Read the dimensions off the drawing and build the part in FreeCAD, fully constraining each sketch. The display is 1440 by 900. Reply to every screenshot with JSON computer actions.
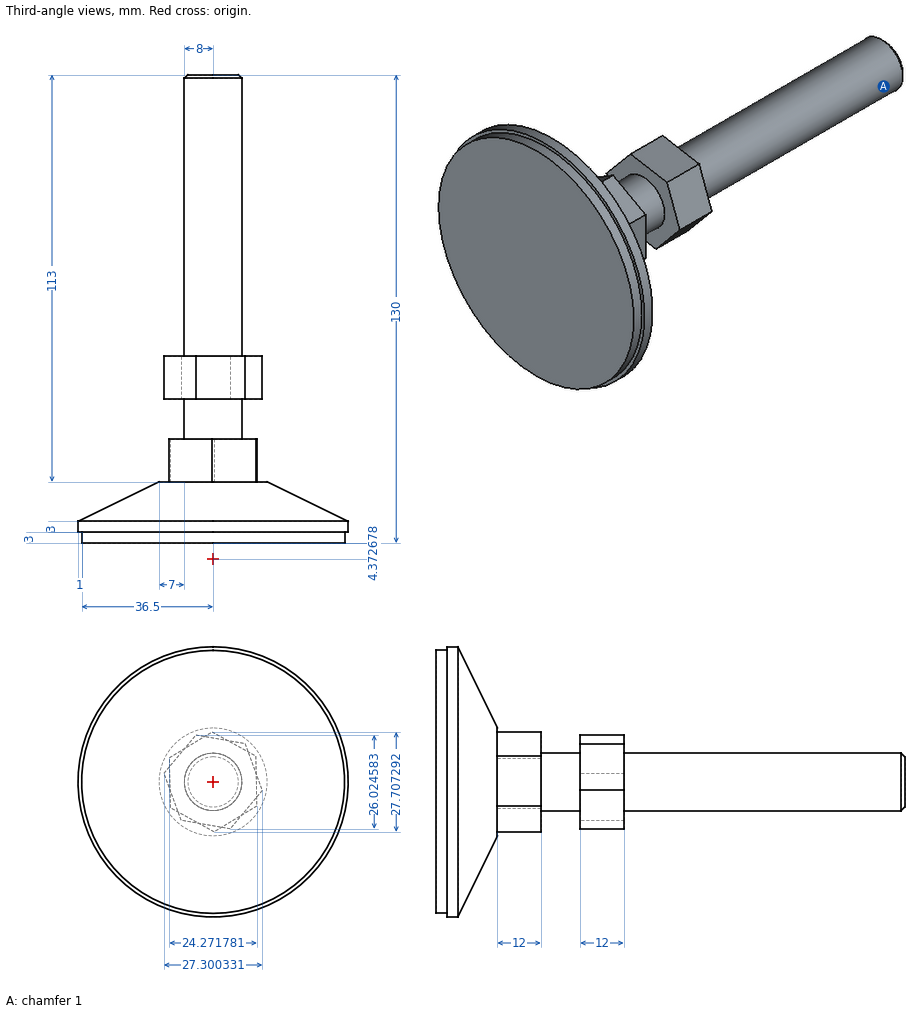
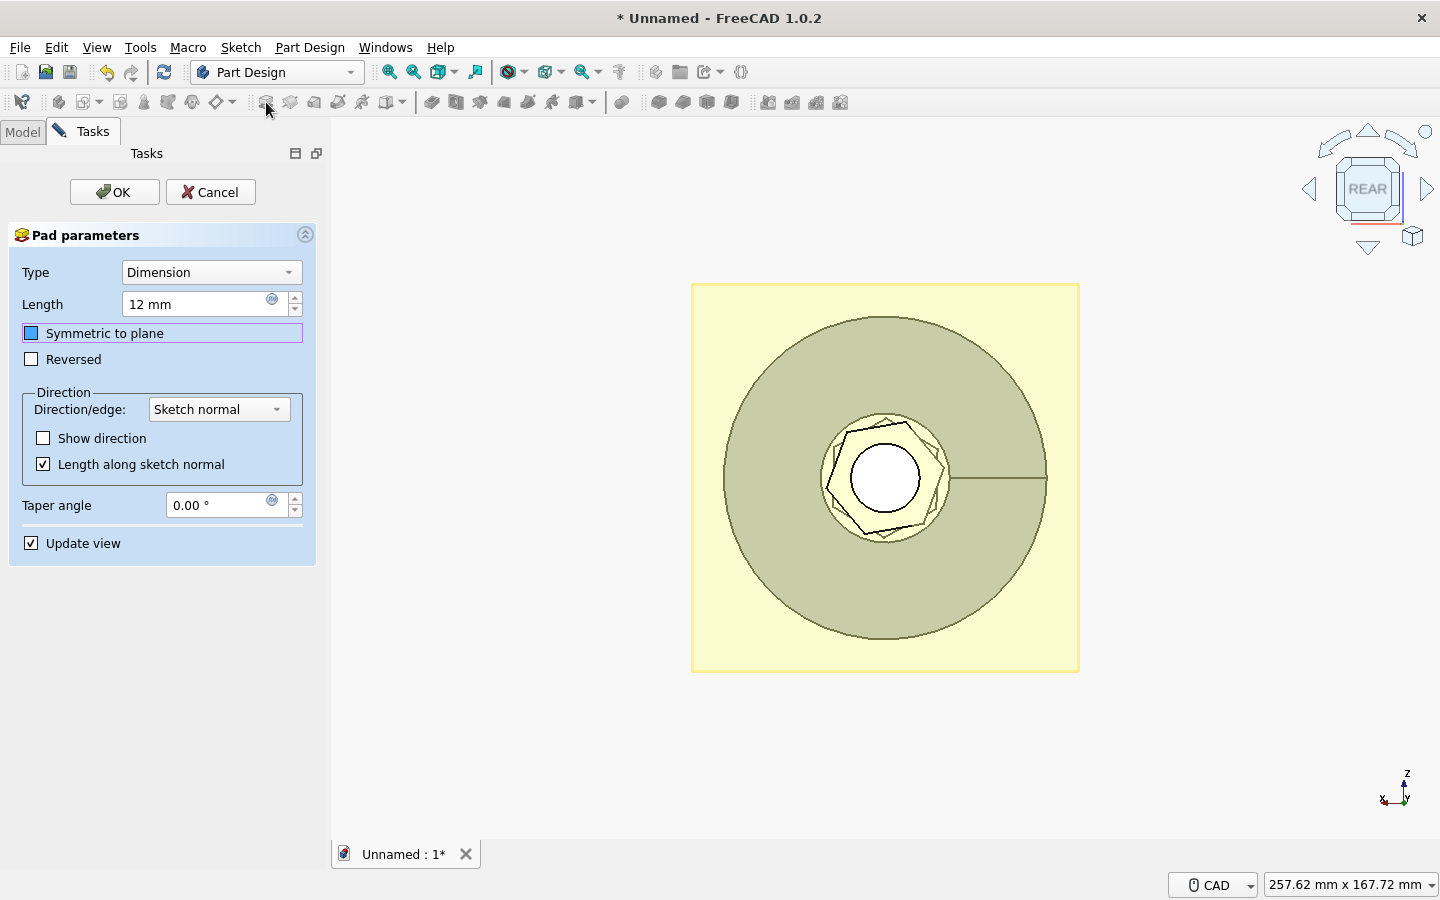
{"action": "left_click", "coordinate": [115, 192]}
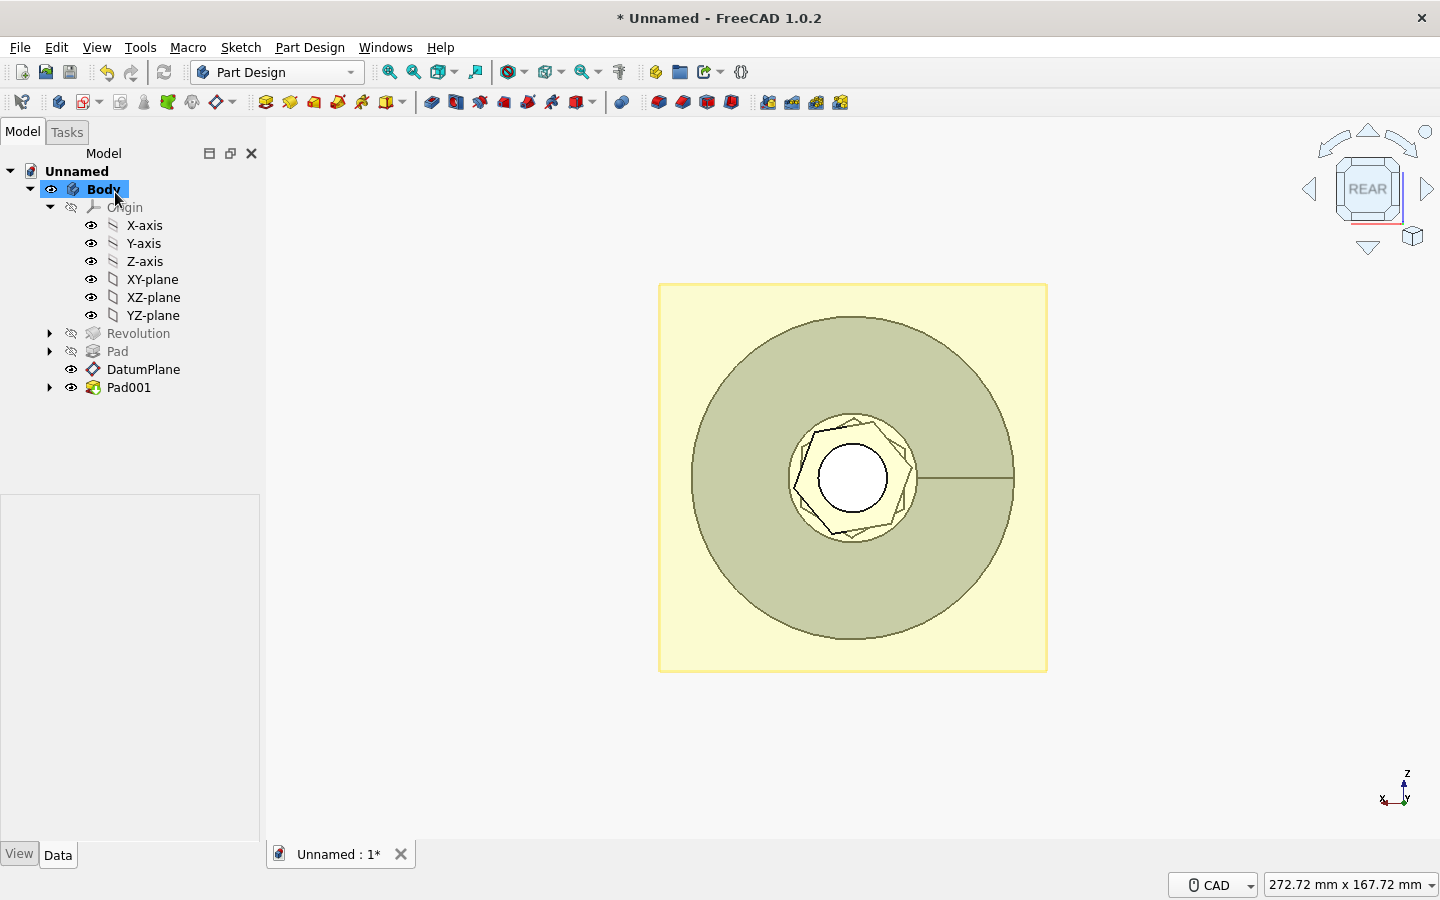
{"action": "left_click", "coordinate": [116, 369]}
{"action": "key", "text": "space"}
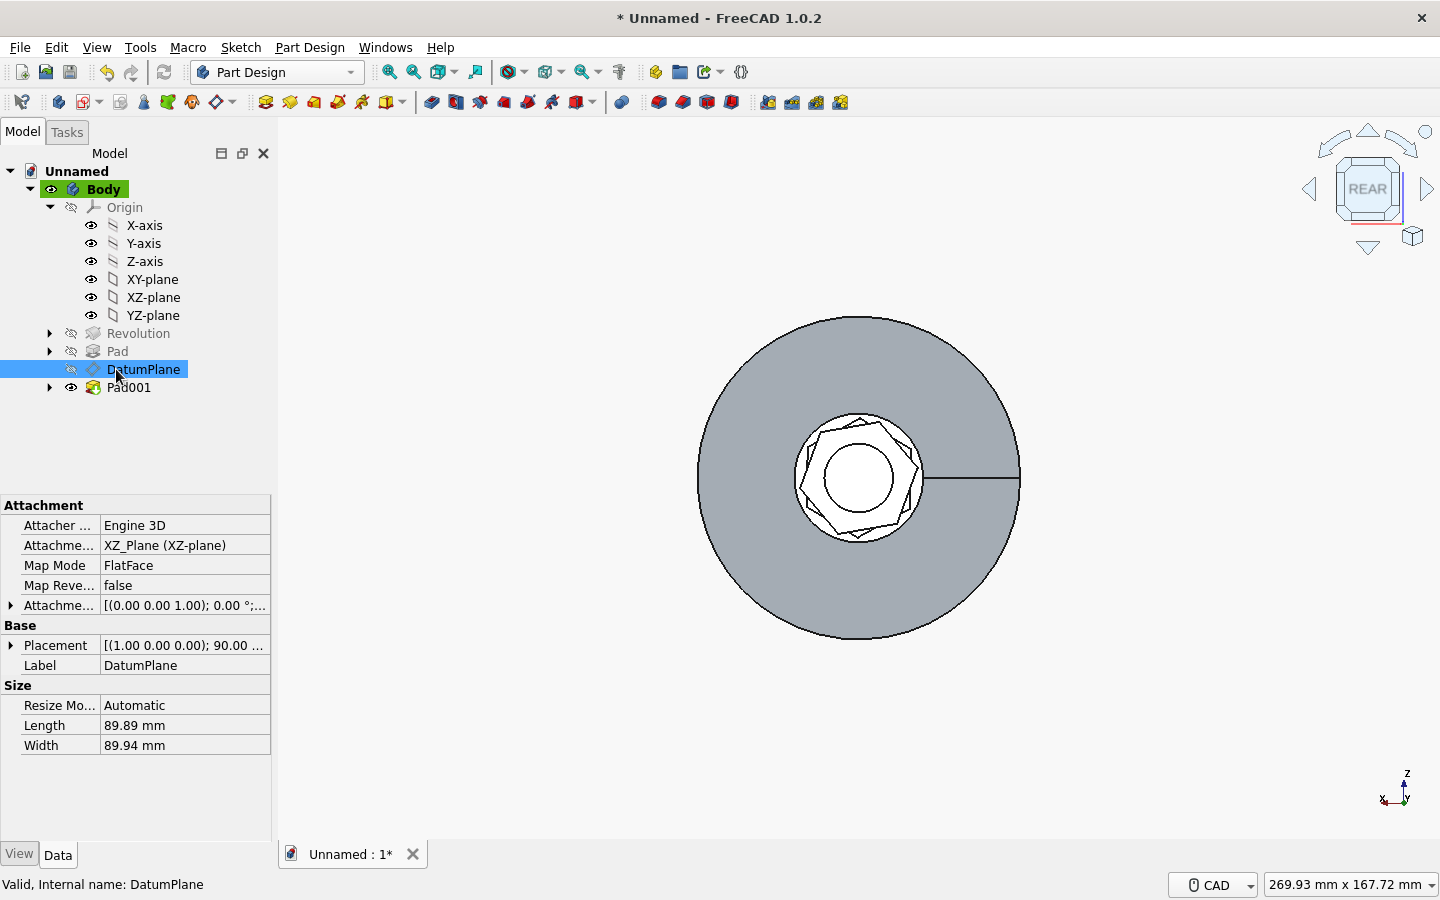
{"action": "left_click", "coordinate": [390, 72]}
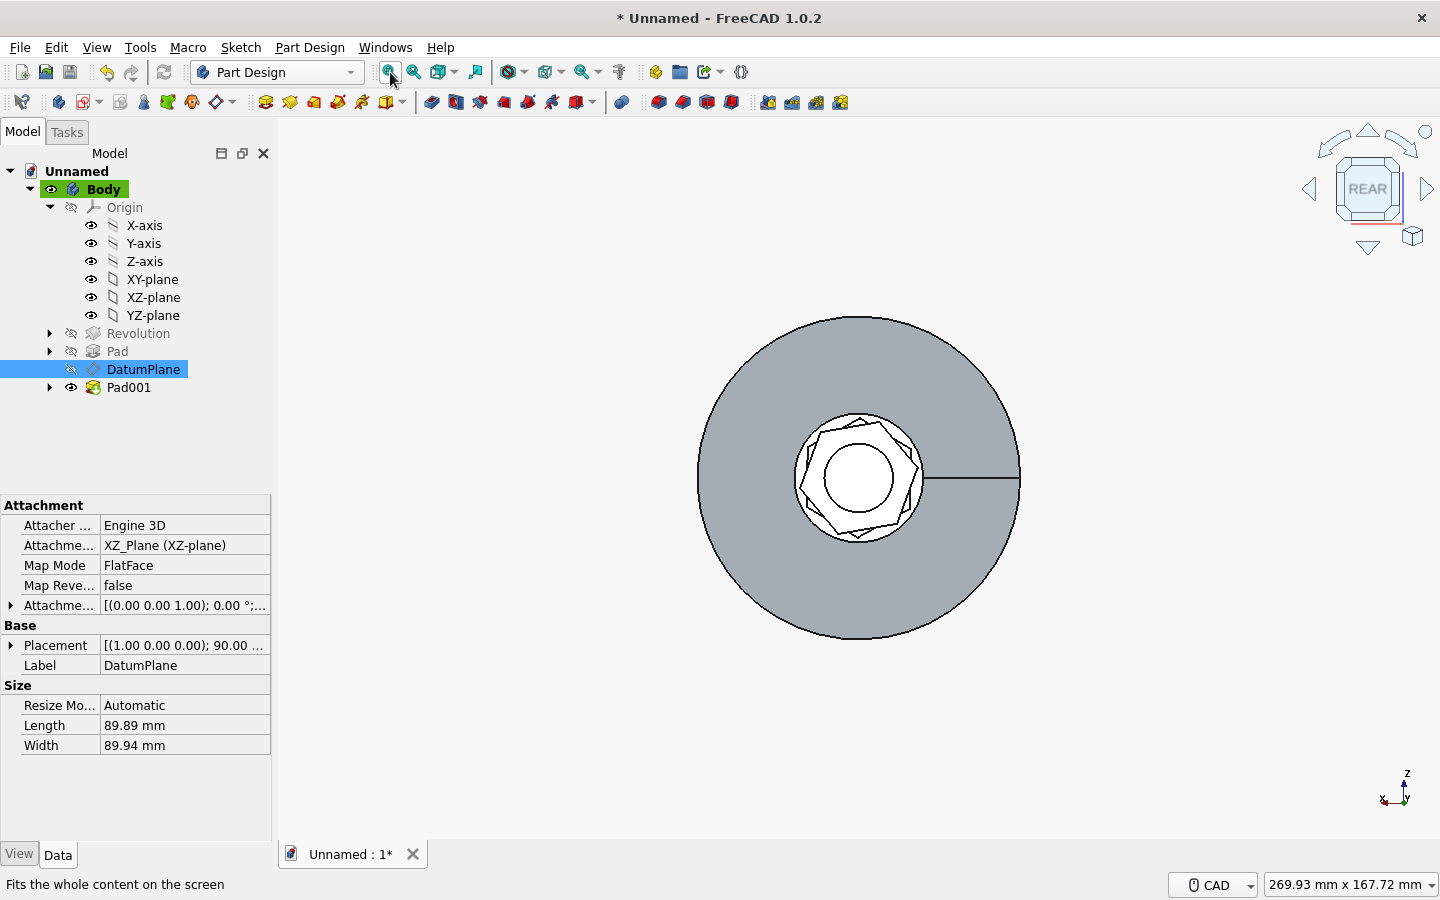
{"action": "left_click", "coordinate": [831, 457]}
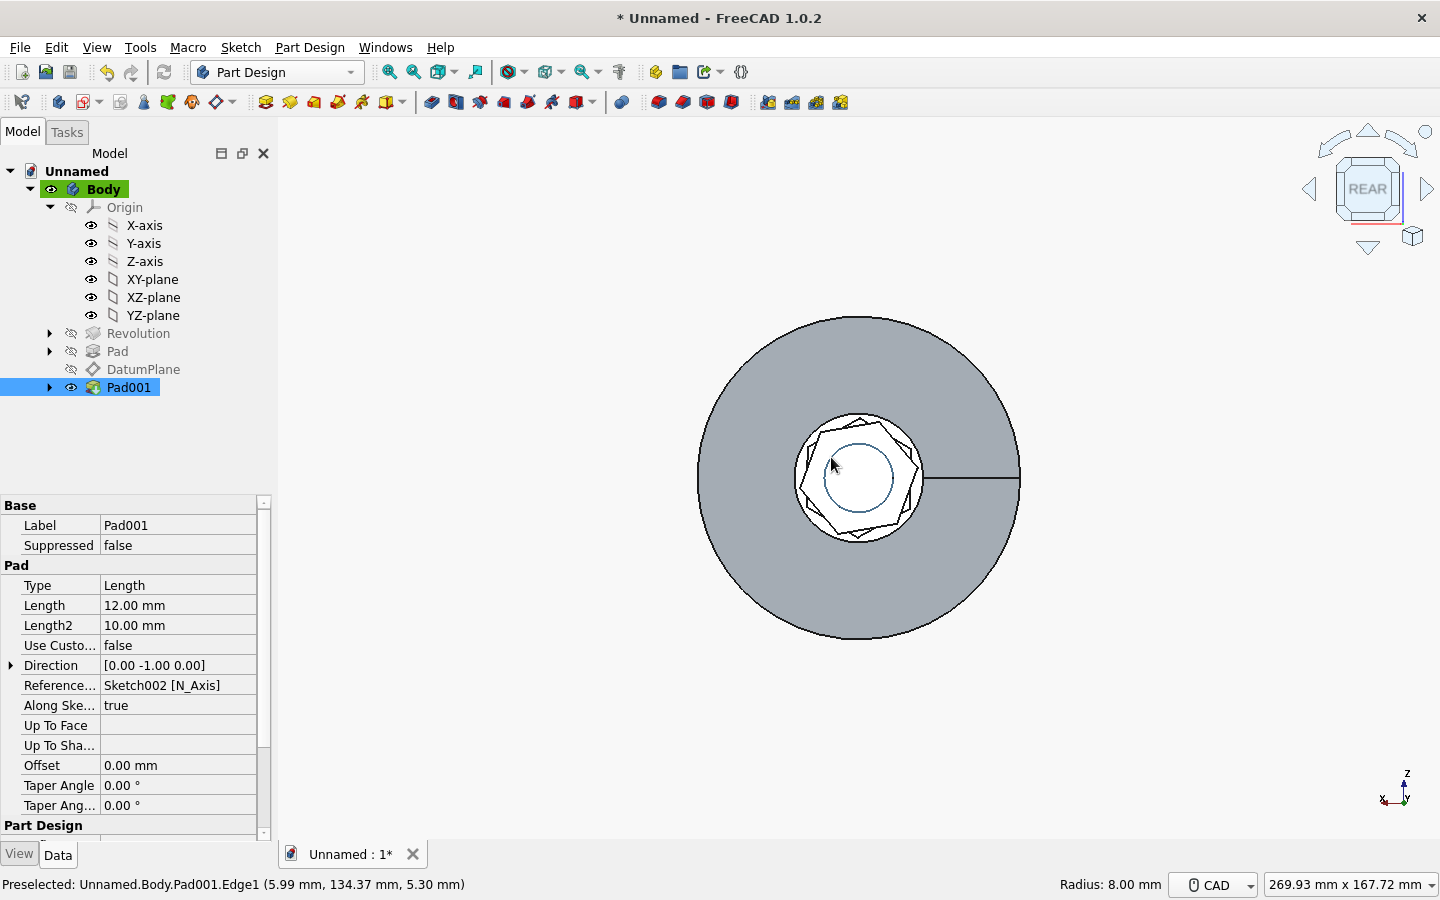
{"action": "left_click", "coordinate": [684, 102]}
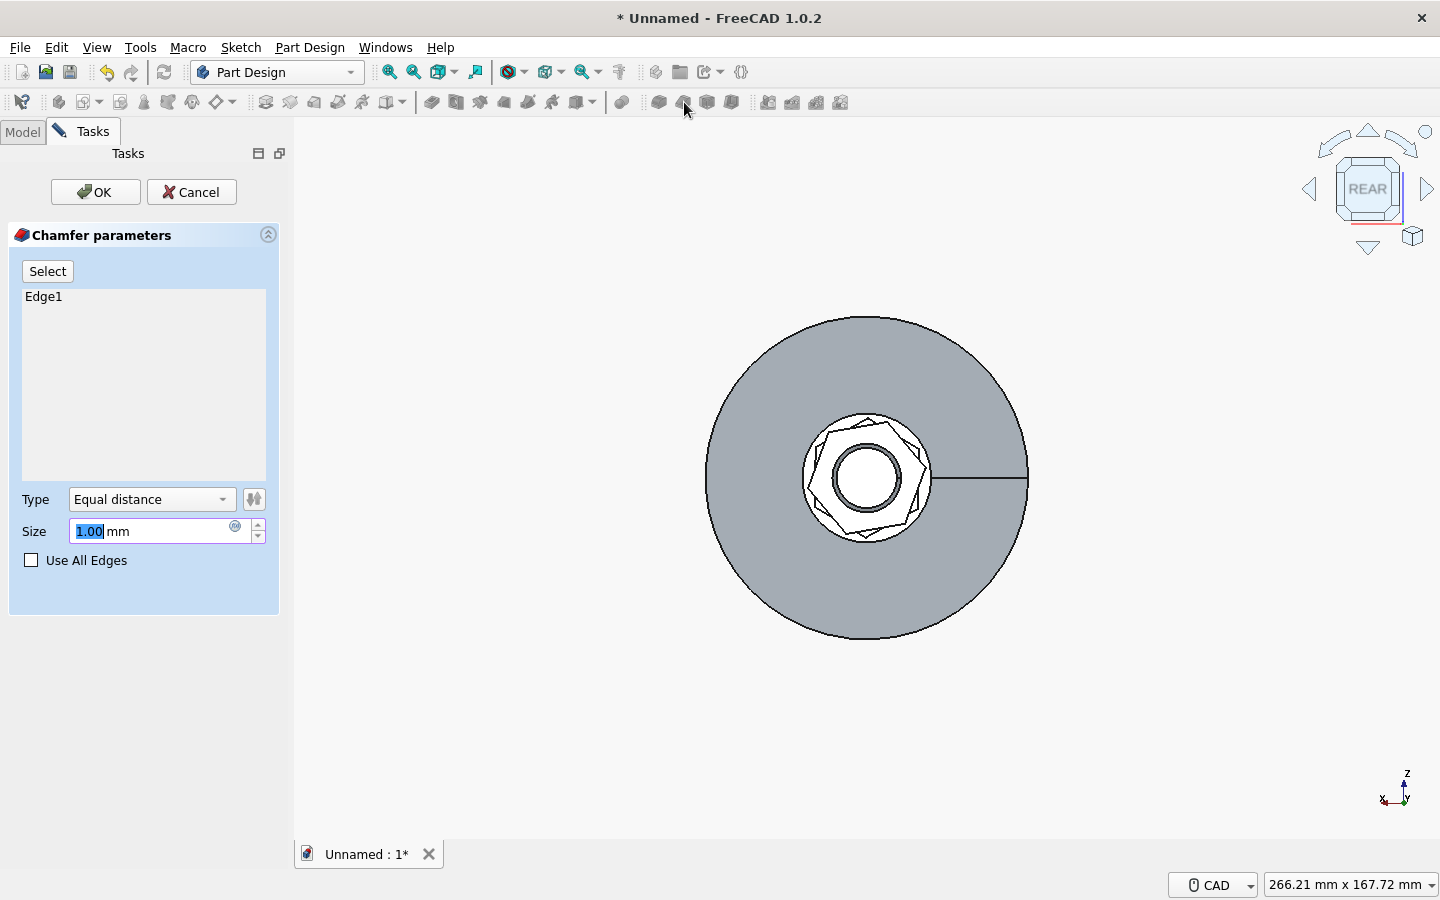
{"action": "type", "text": "1"}
{"action": "key", "text": "Tab"}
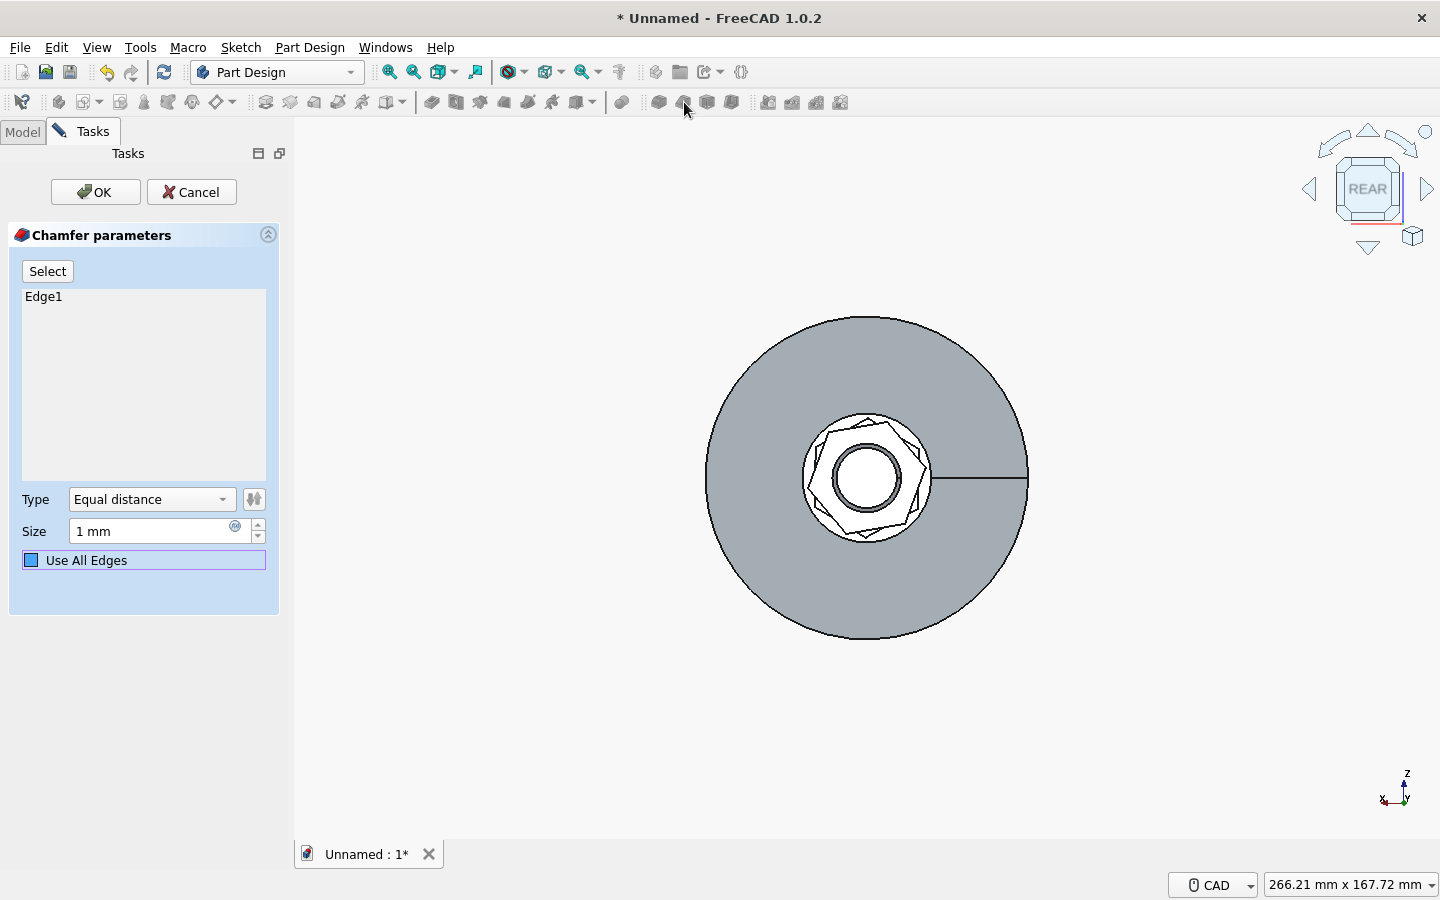
{"action": "left_click", "coordinate": [96, 192]}